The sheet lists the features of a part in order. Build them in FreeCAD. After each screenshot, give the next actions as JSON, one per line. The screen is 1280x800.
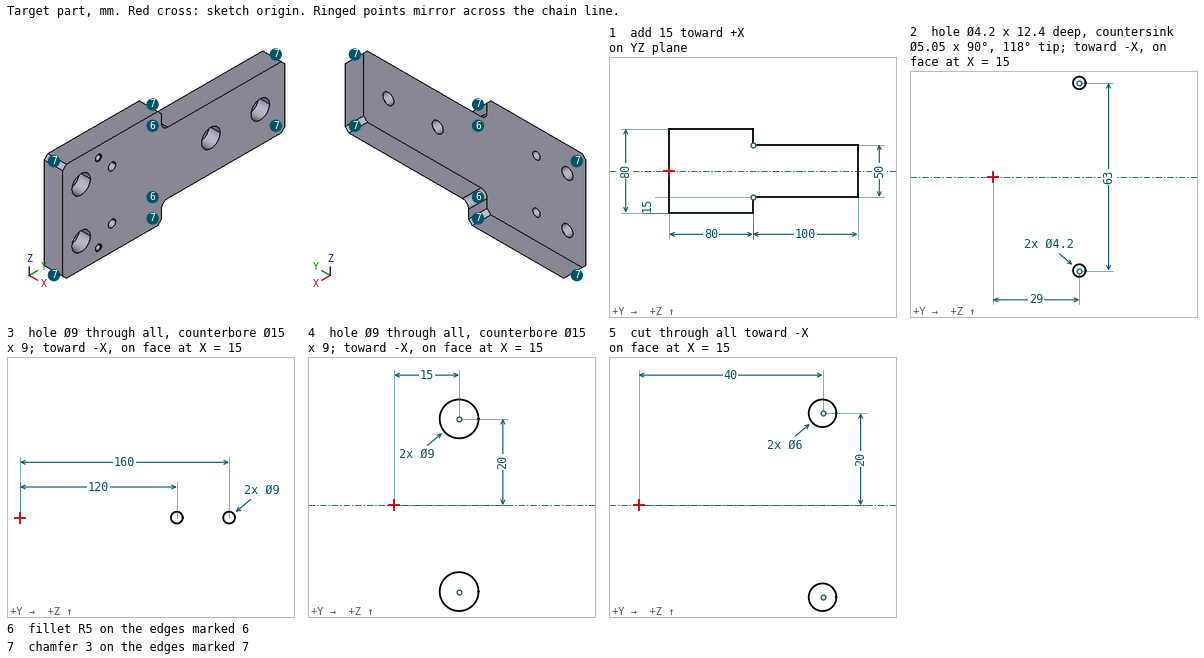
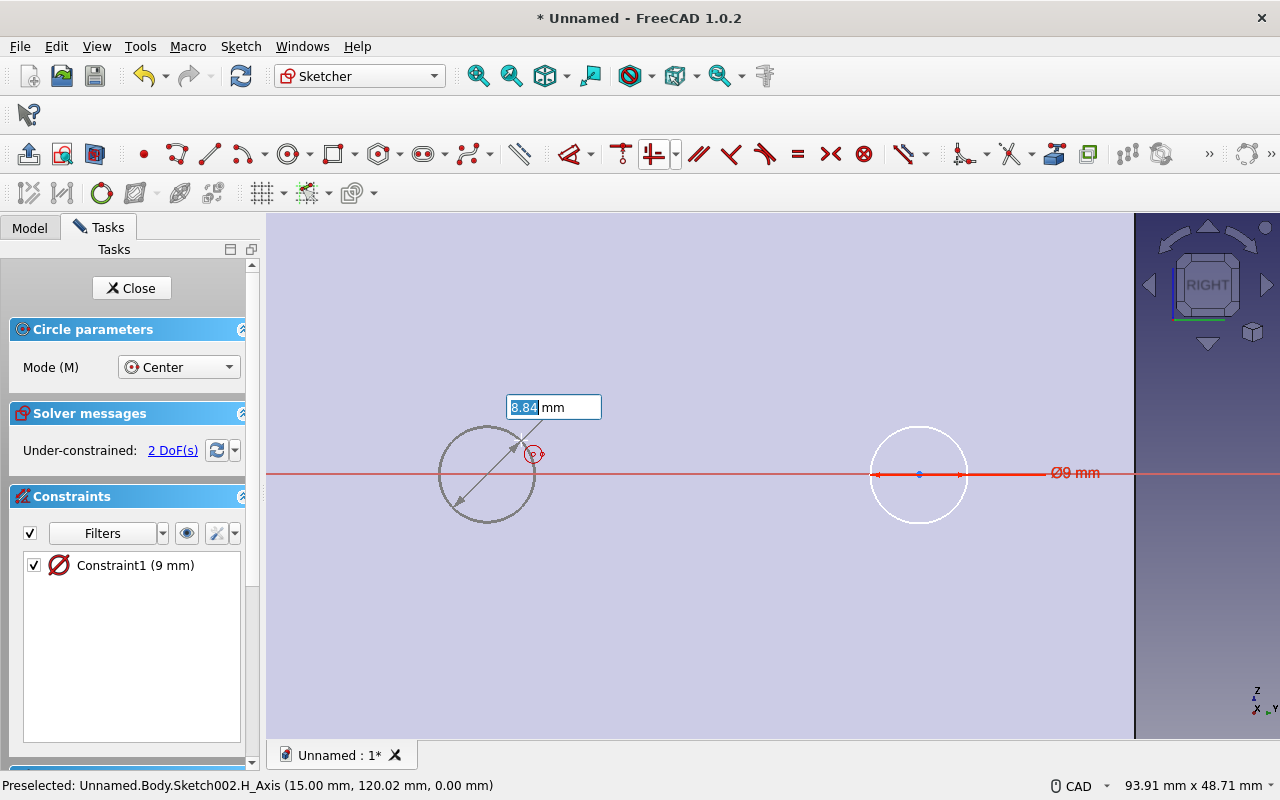
{"action": "type", "text": "9"}
{"action": "key", "text": "Return"}
{"action": "key", "text": "Escape"}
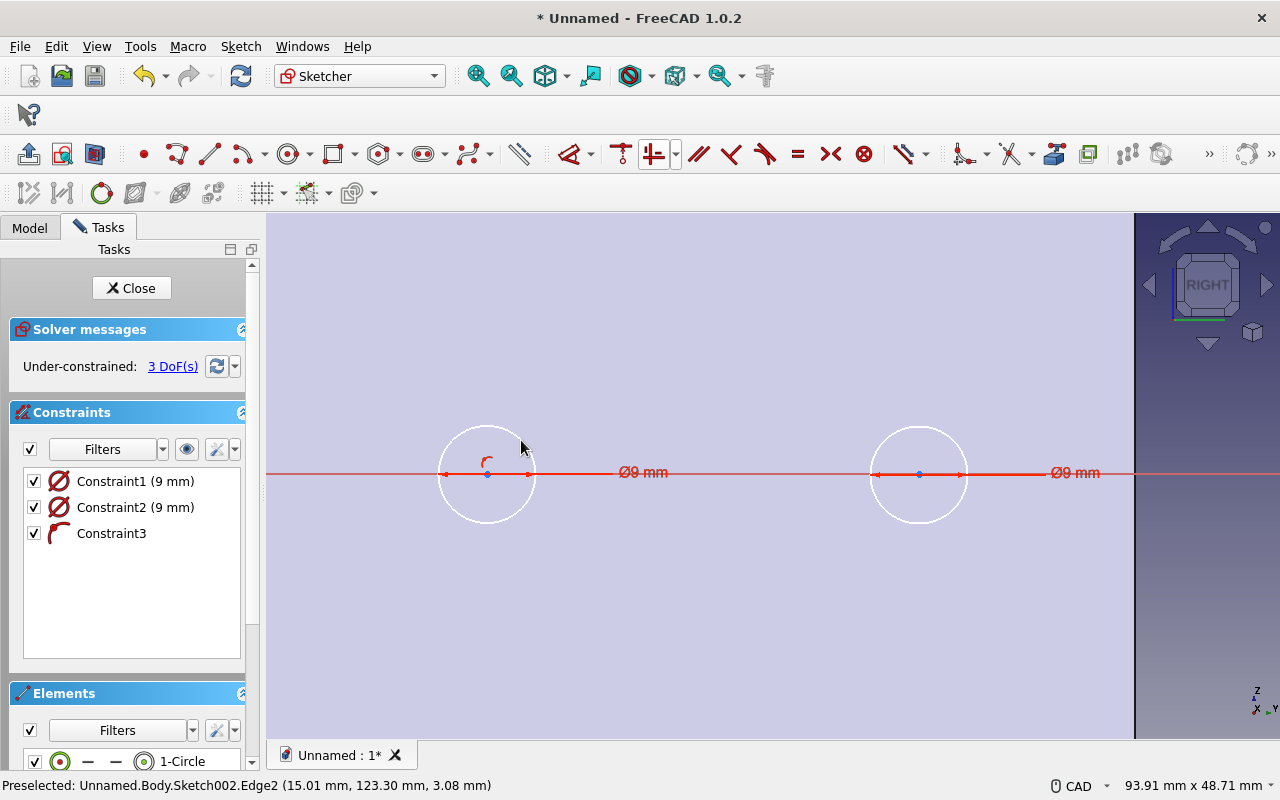
{"action": "left_click", "coordinate": [919, 475]}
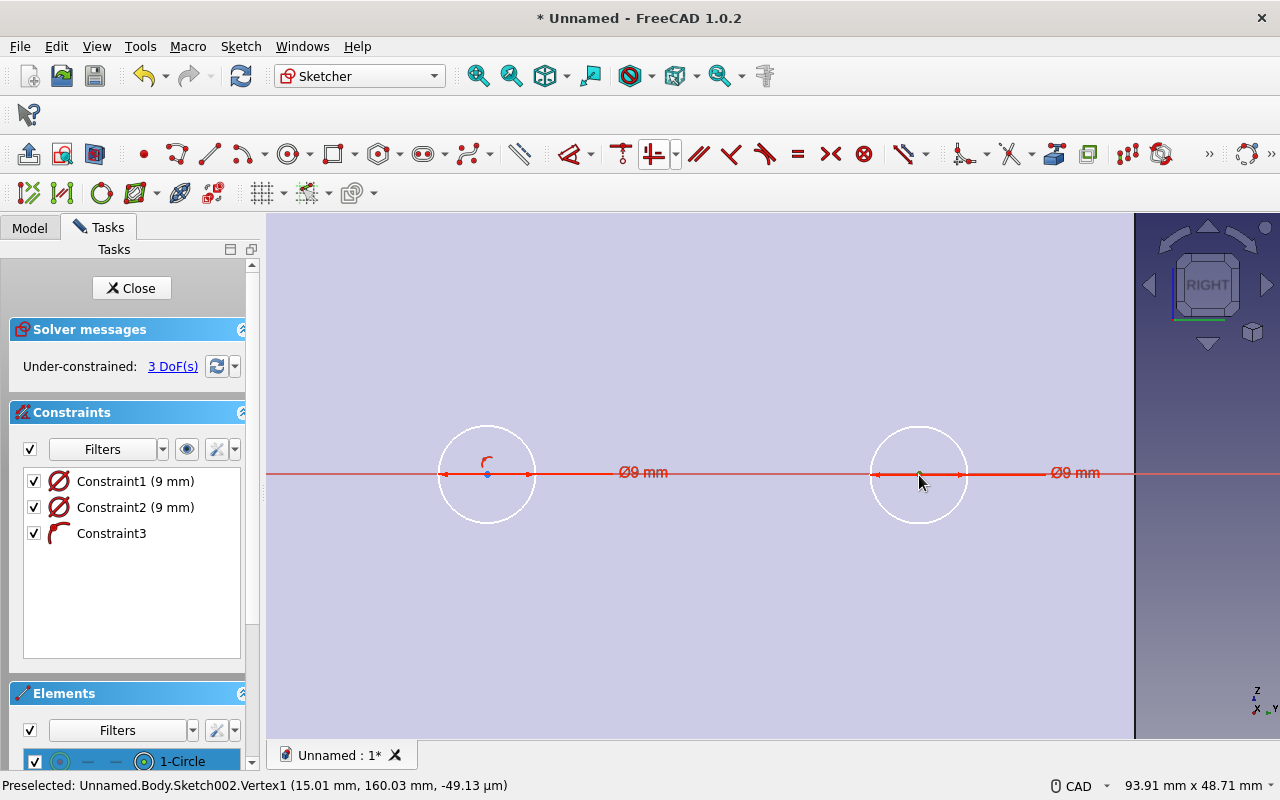
{"action": "left_click", "coordinate": [353, 474]}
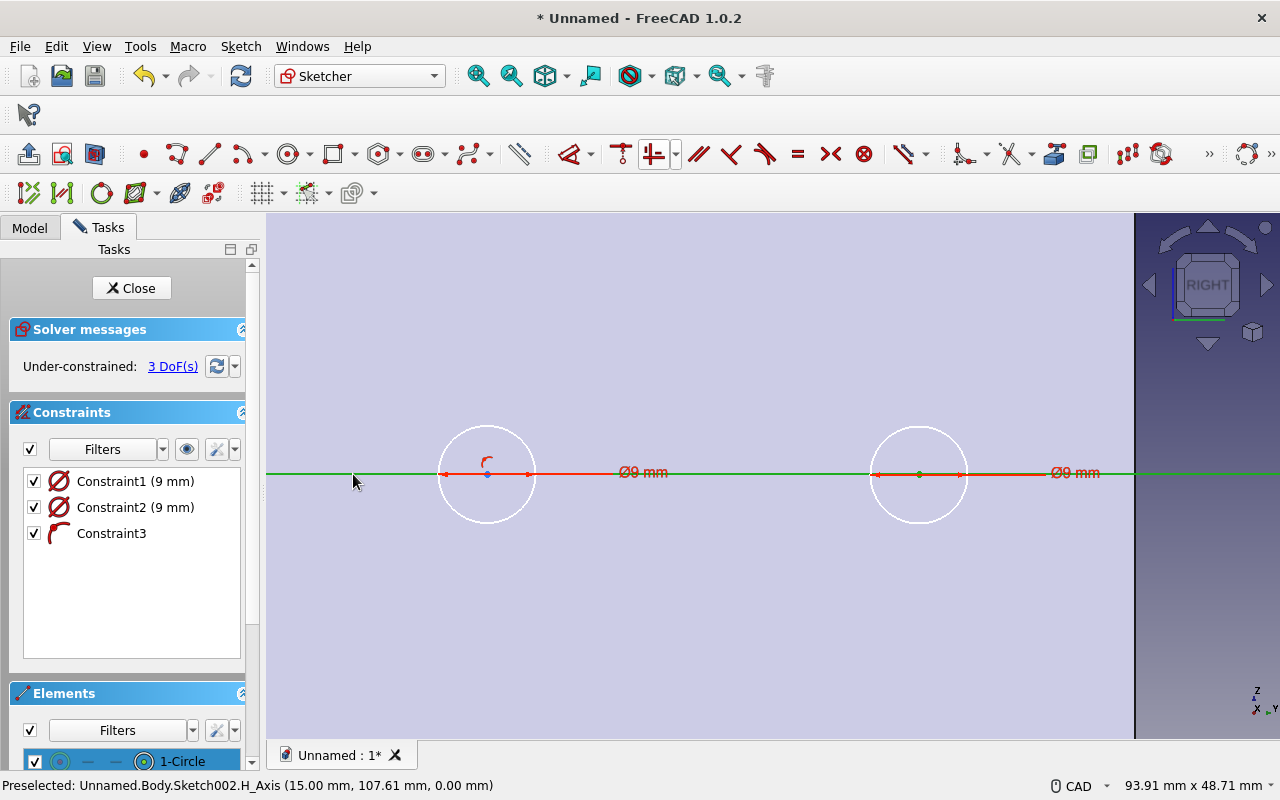
{"action": "left_click", "coordinate": [621, 154]}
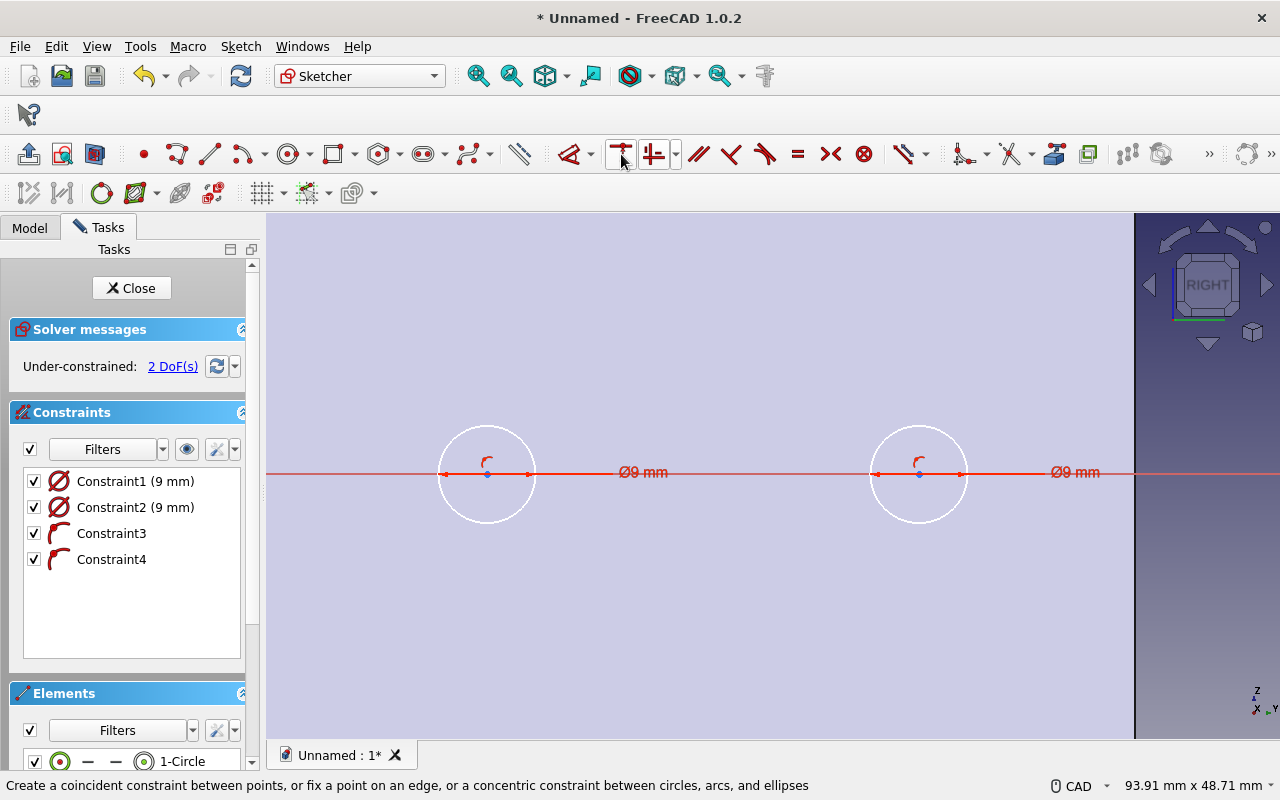
{"action": "left_click", "coordinate": [568, 154]}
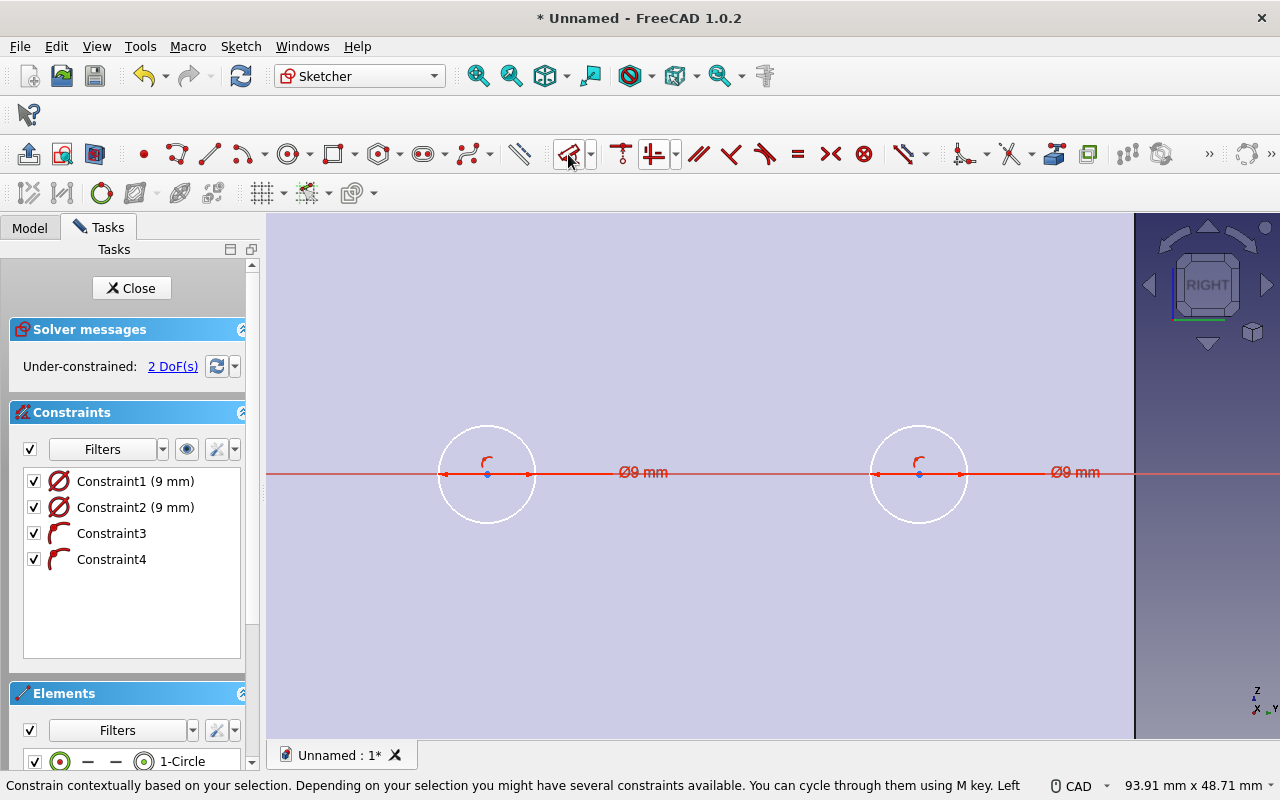
{"action": "left_click", "coordinate": [919, 474]}
{"action": "left_click", "coordinate": [607, 508]}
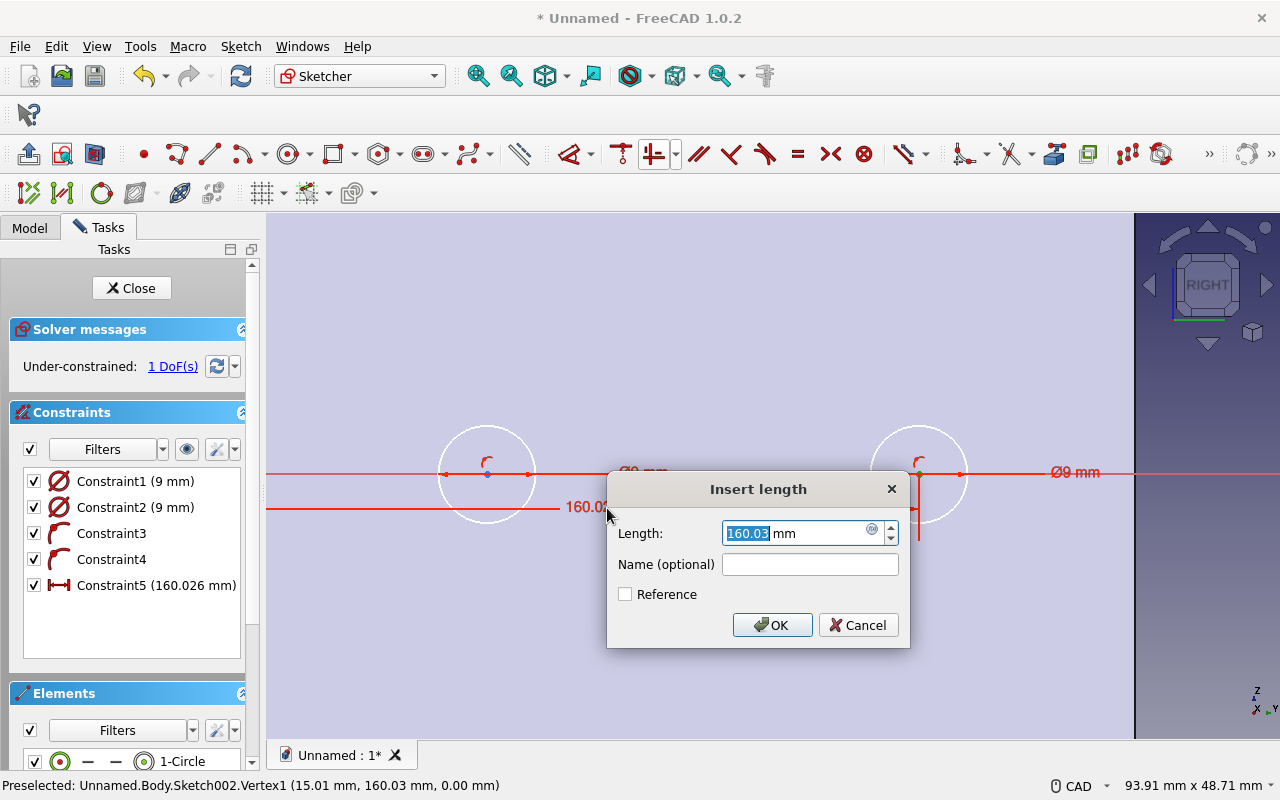
{"action": "type", "text": "160"}
{"action": "key", "text": "Return"}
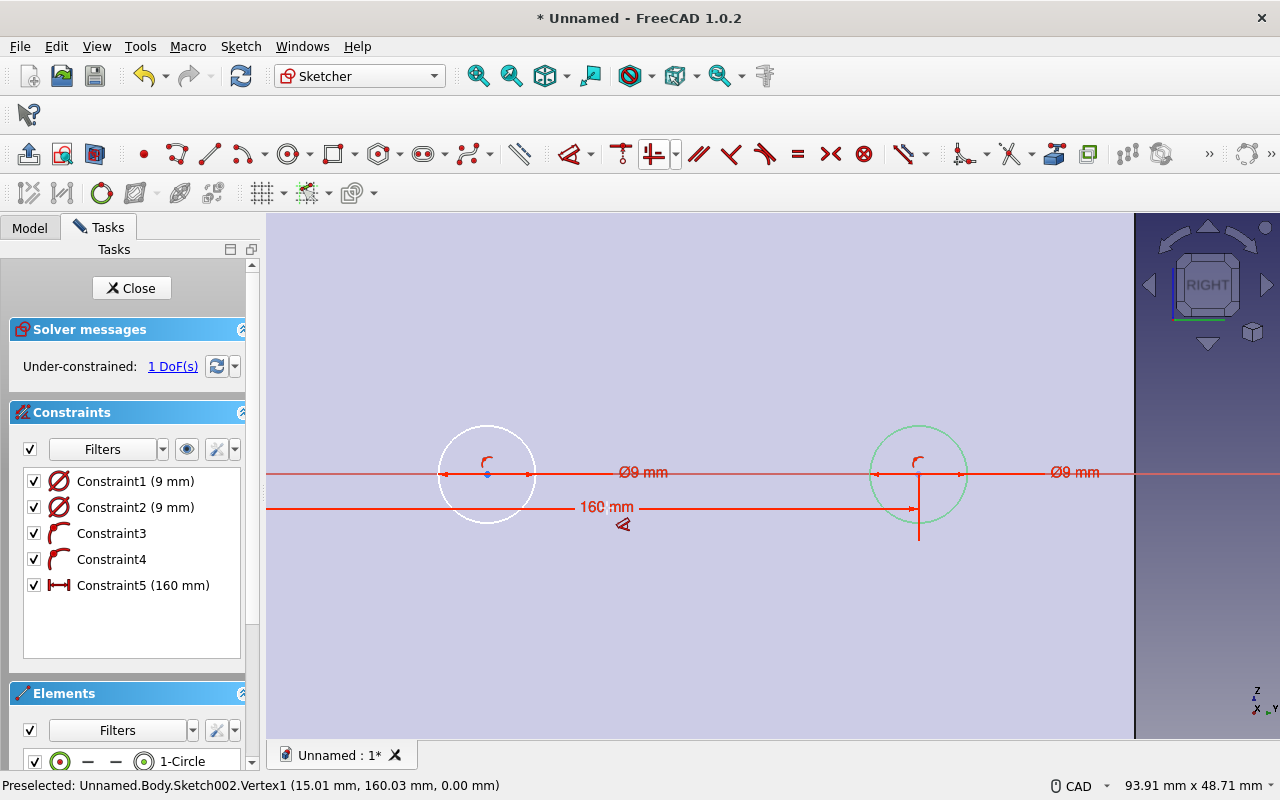
{"action": "left_click", "coordinate": [487, 474]}
{"action": "left_click", "coordinate": [390, 508]}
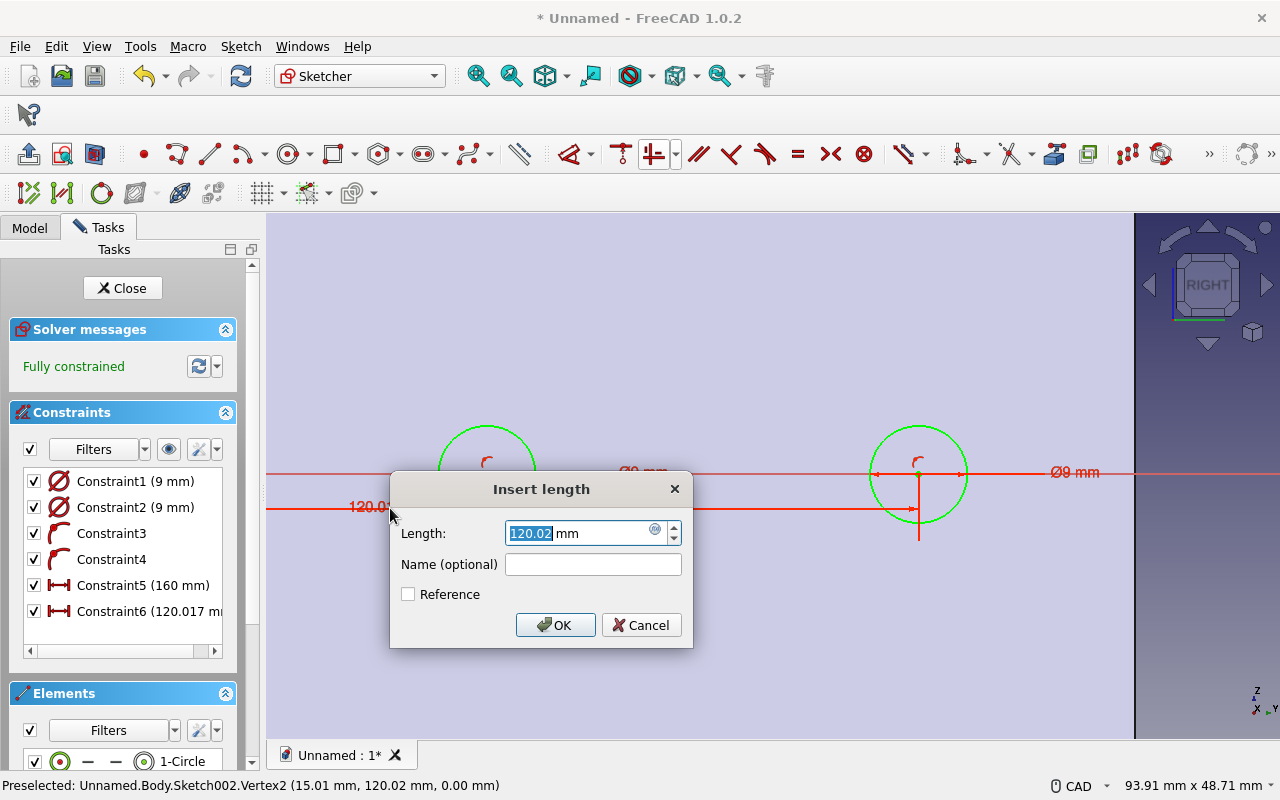
{"action": "type", "text": "120"}
{"action": "key", "text": "Return"}
{"action": "key", "text": "Escape"}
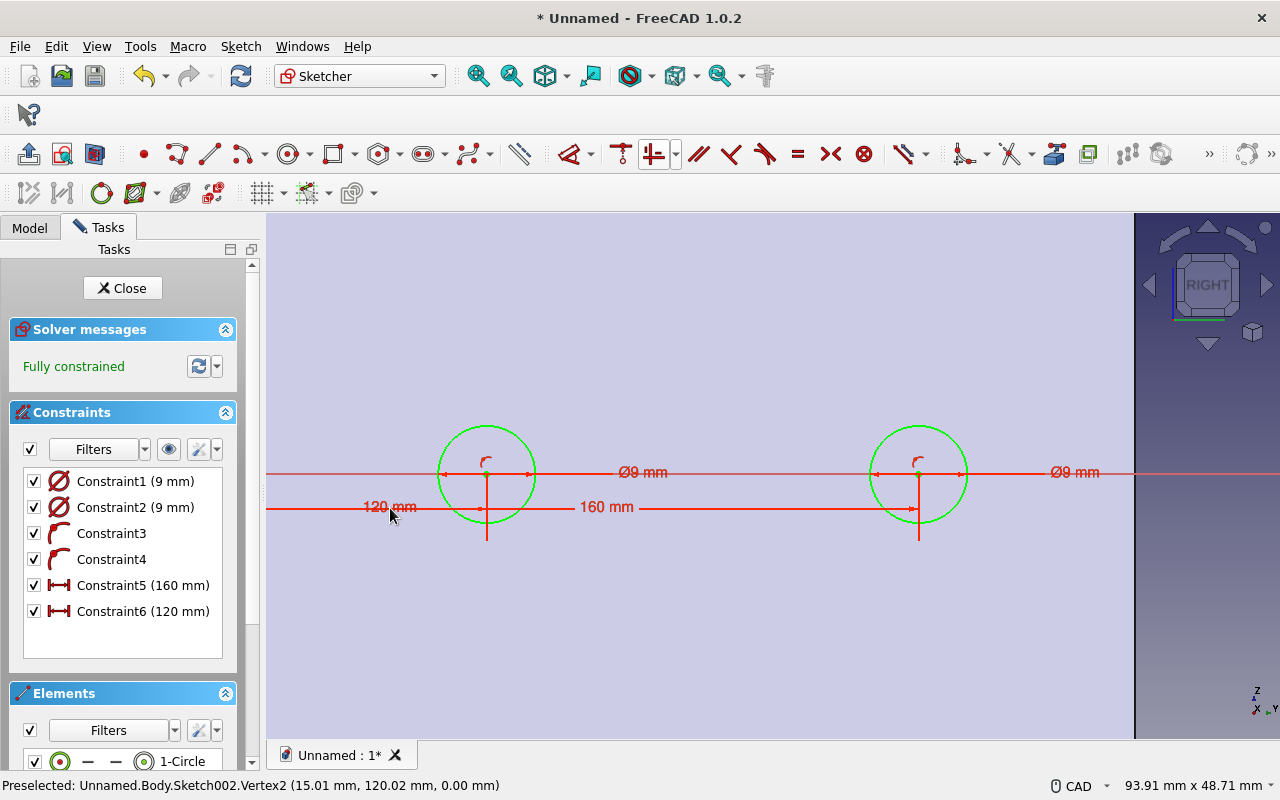
{"action": "left_click", "coordinate": [123, 288]}